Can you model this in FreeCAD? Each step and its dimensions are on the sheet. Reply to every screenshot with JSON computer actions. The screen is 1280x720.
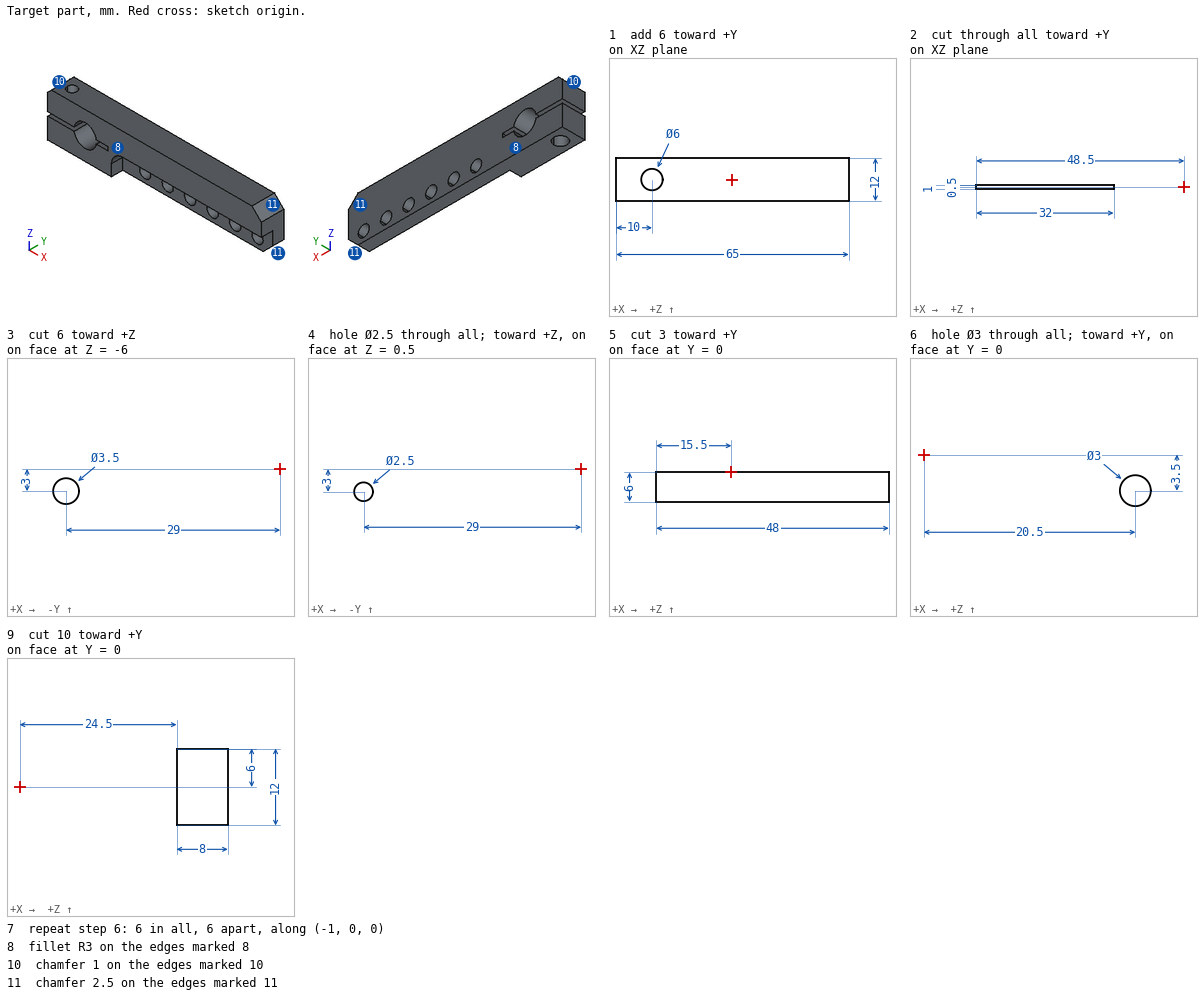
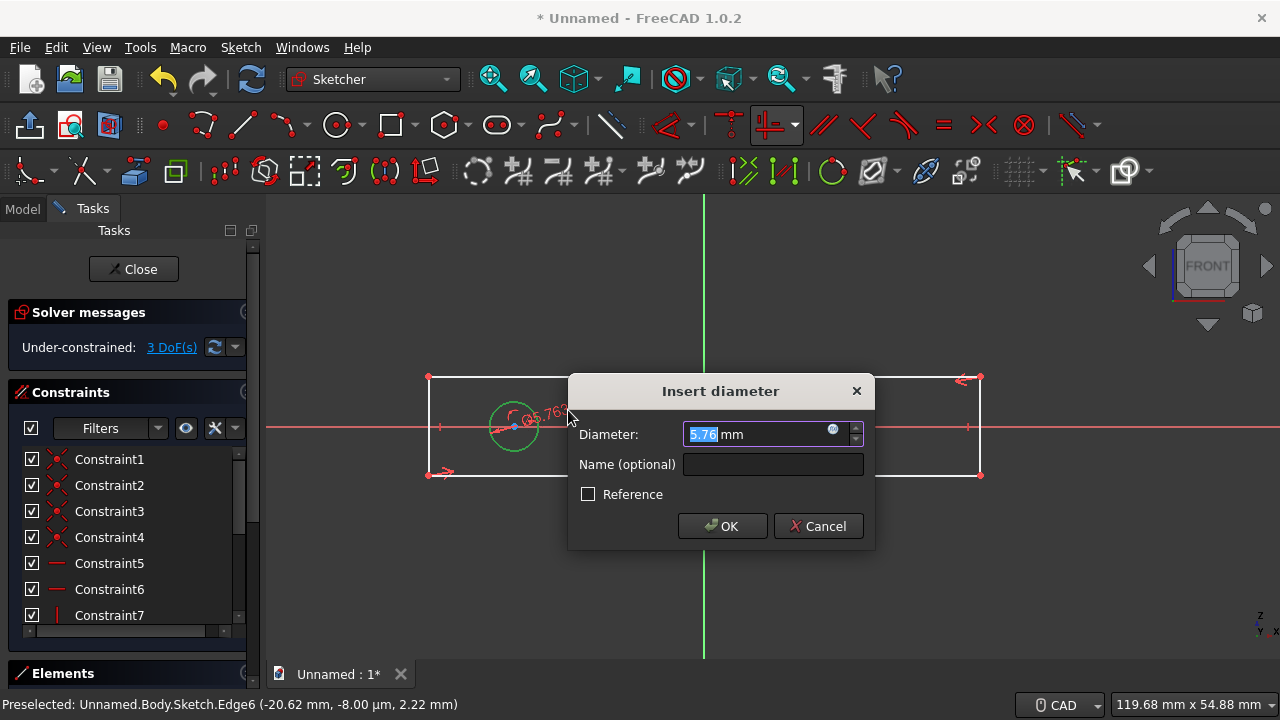
{"action": "type", "text": "6"}
{"action": "key", "text": "Return"}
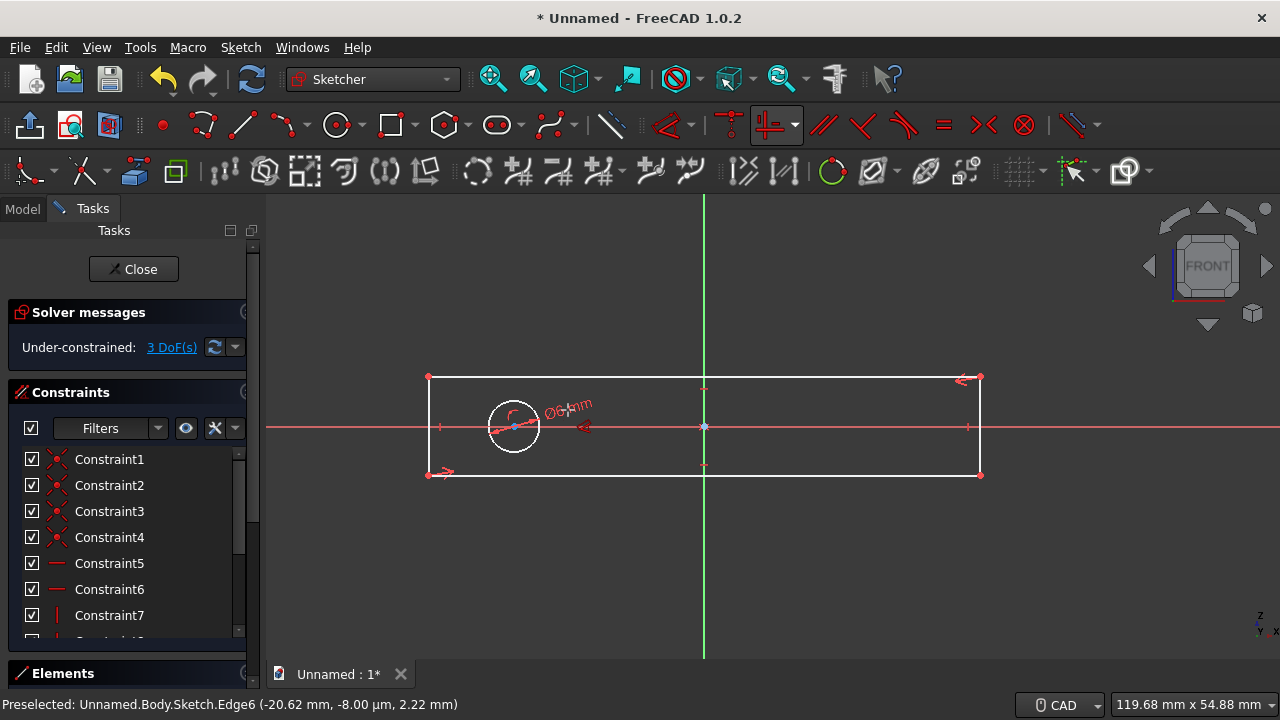
{"action": "left_click", "coordinate": [594, 476]}
{"action": "left_click", "coordinate": [577, 510]}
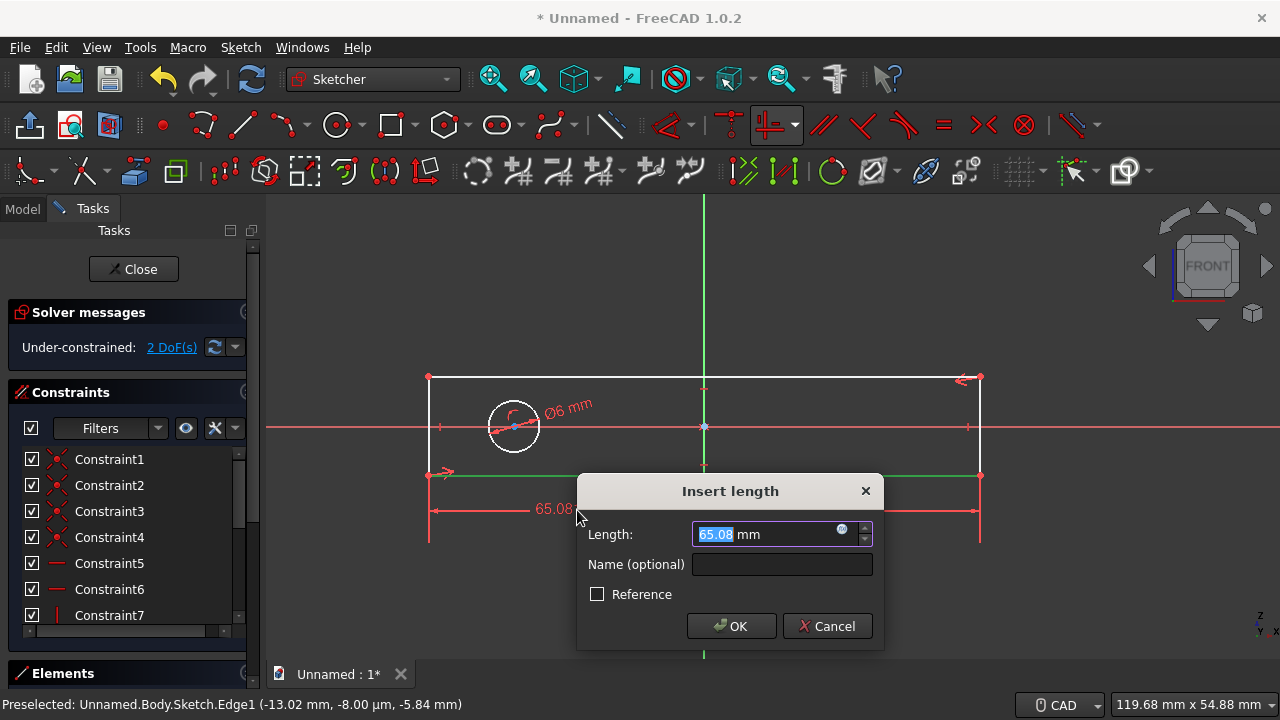
{"action": "type", "text": "65"}
{"action": "key", "text": "Return"}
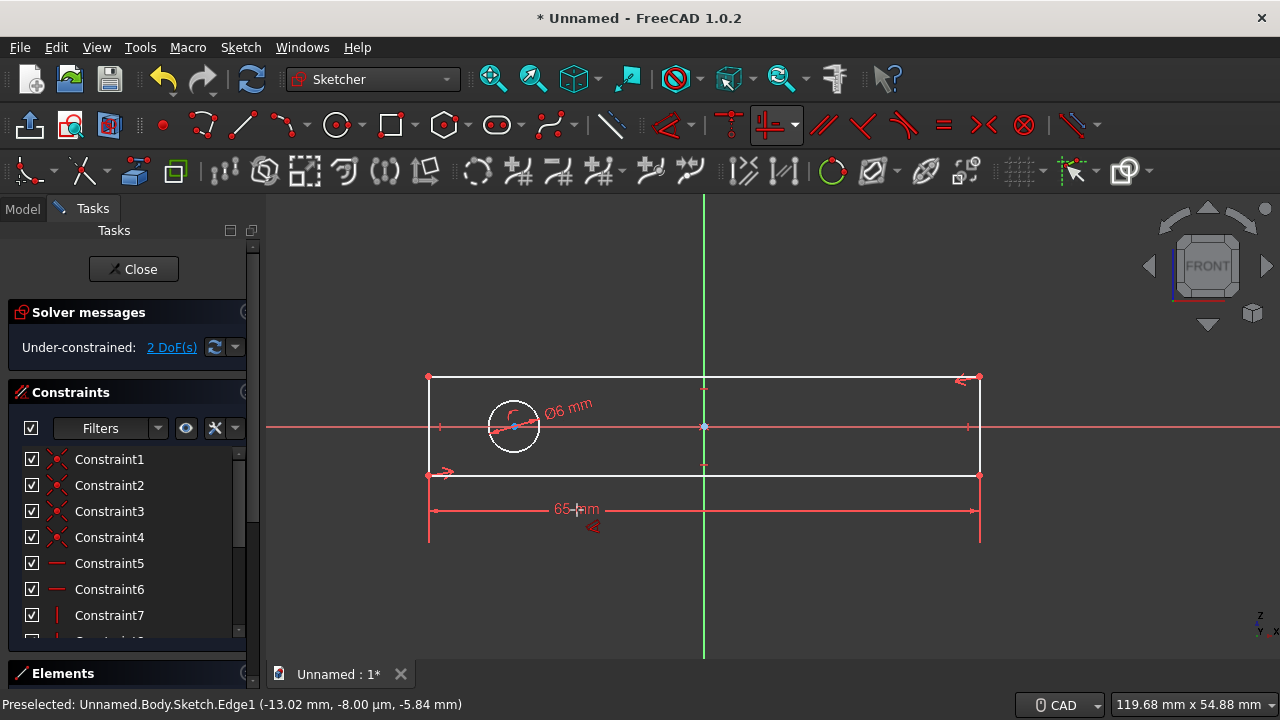
{"action": "left_click", "coordinate": [980, 446]}
{"action": "left_click", "coordinate": [1014, 404]}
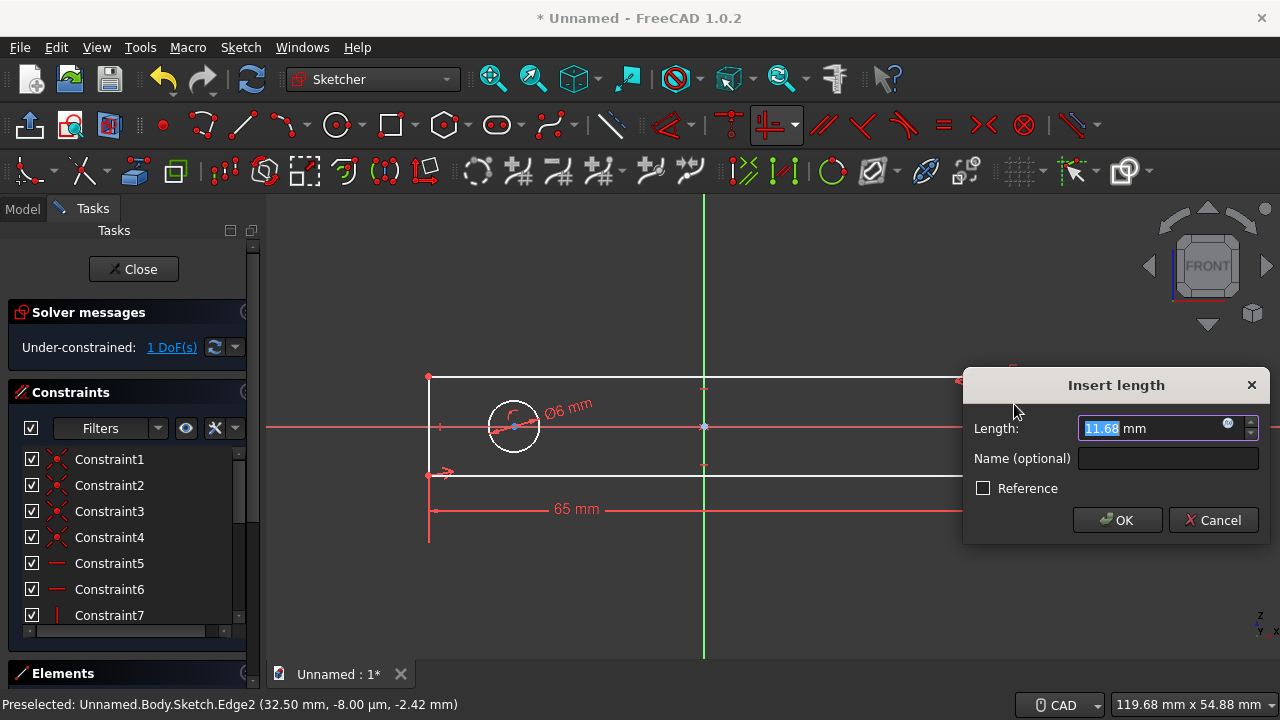
{"action": "type", "text": "12"}
{"action": "key", "text": "Return"}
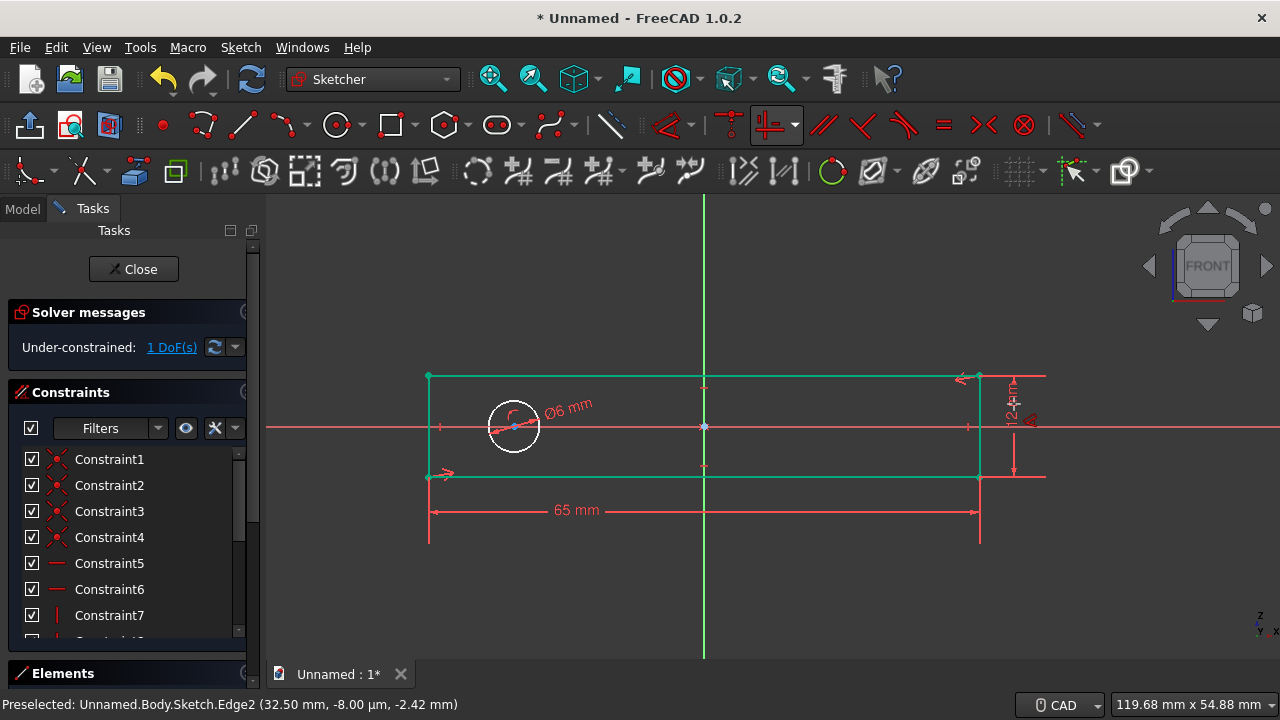
{"action": "left_click", "coordinate": [429, 477]}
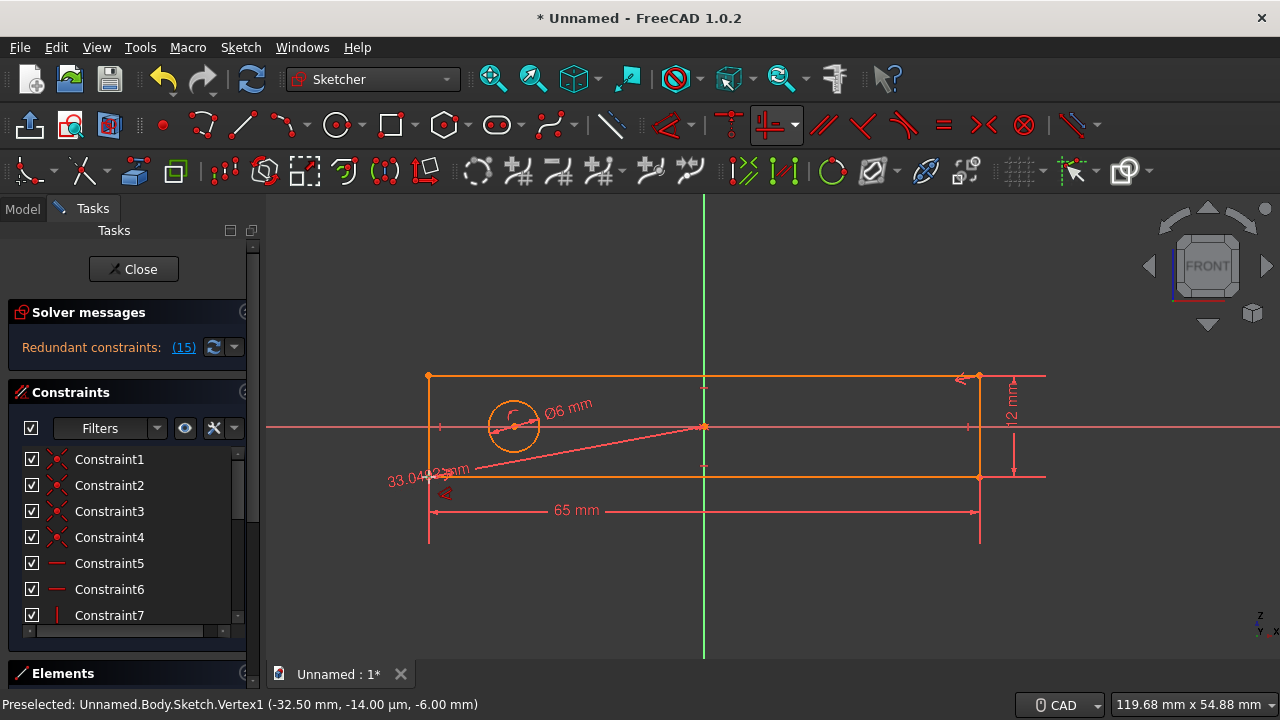
{"action": "left_click", "coordinate": [514, 426]}
{"action": "left_click", "coordinate": [471, 511]}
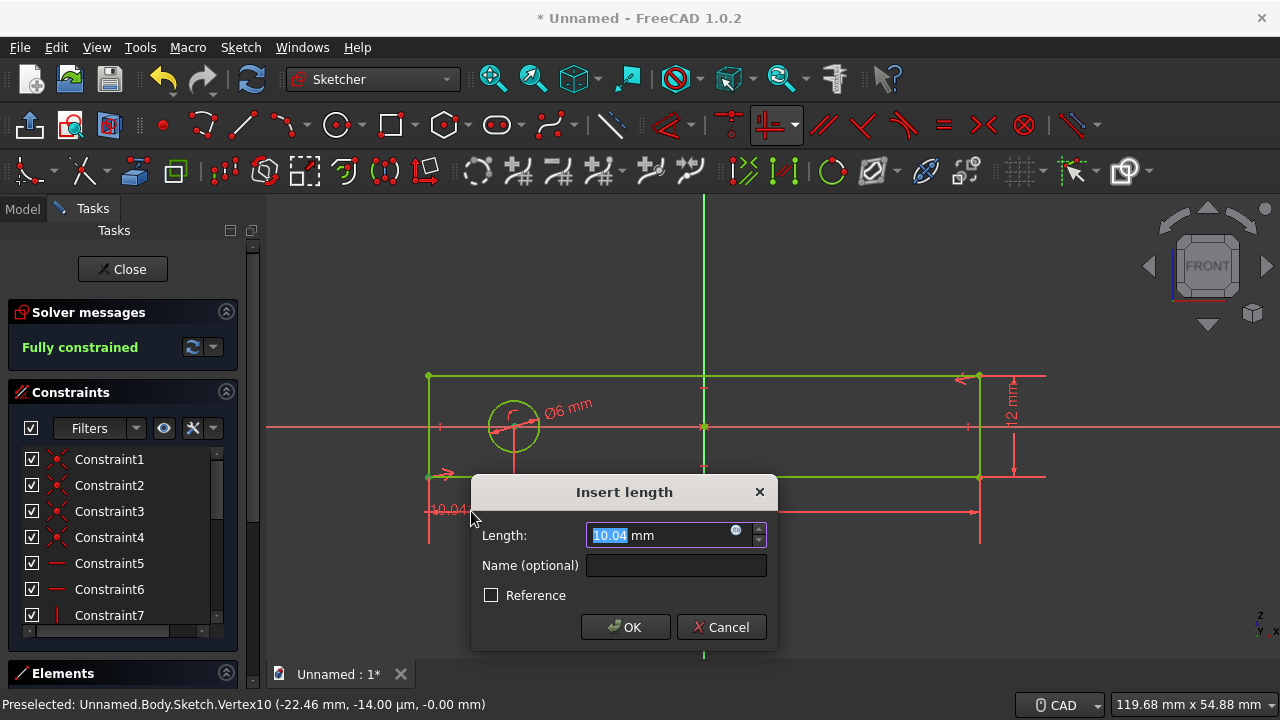
{"action": "type", "text": "10"}
{"action": "key", "text": "Return"}
{"action": "key", "text": "Escape"}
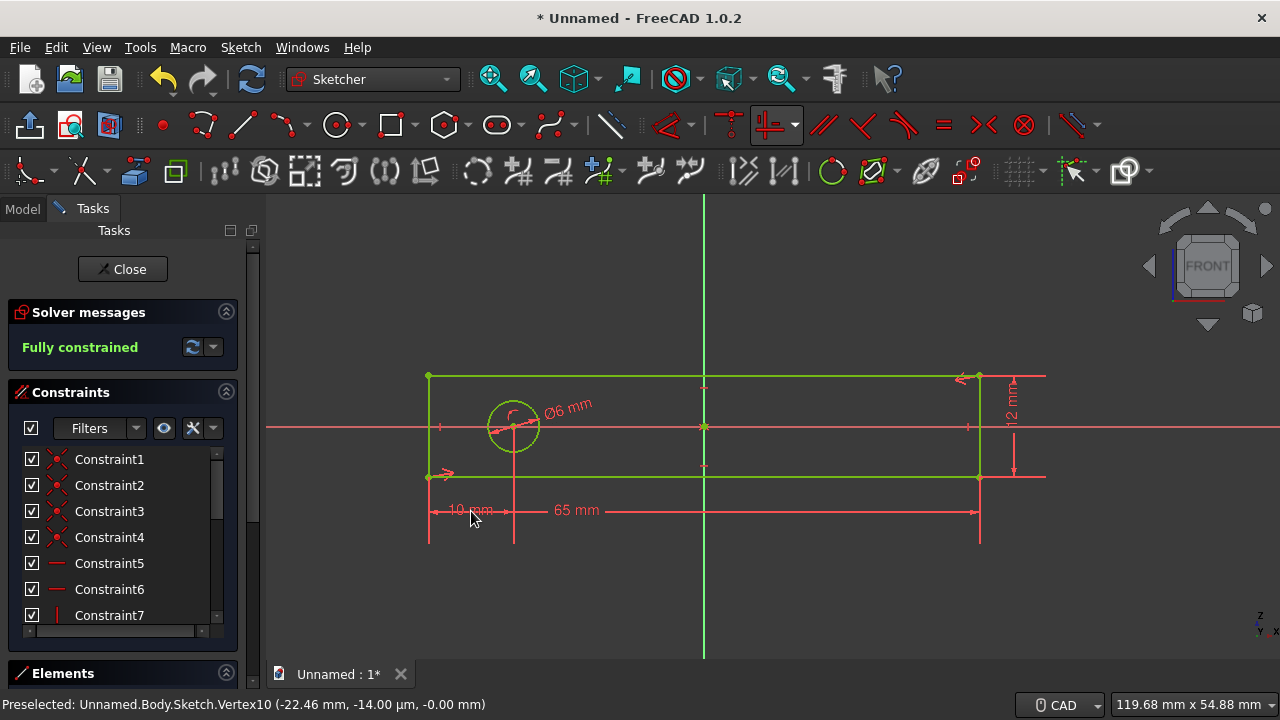
{"action": "left_click", "coordinate": [123, 269]}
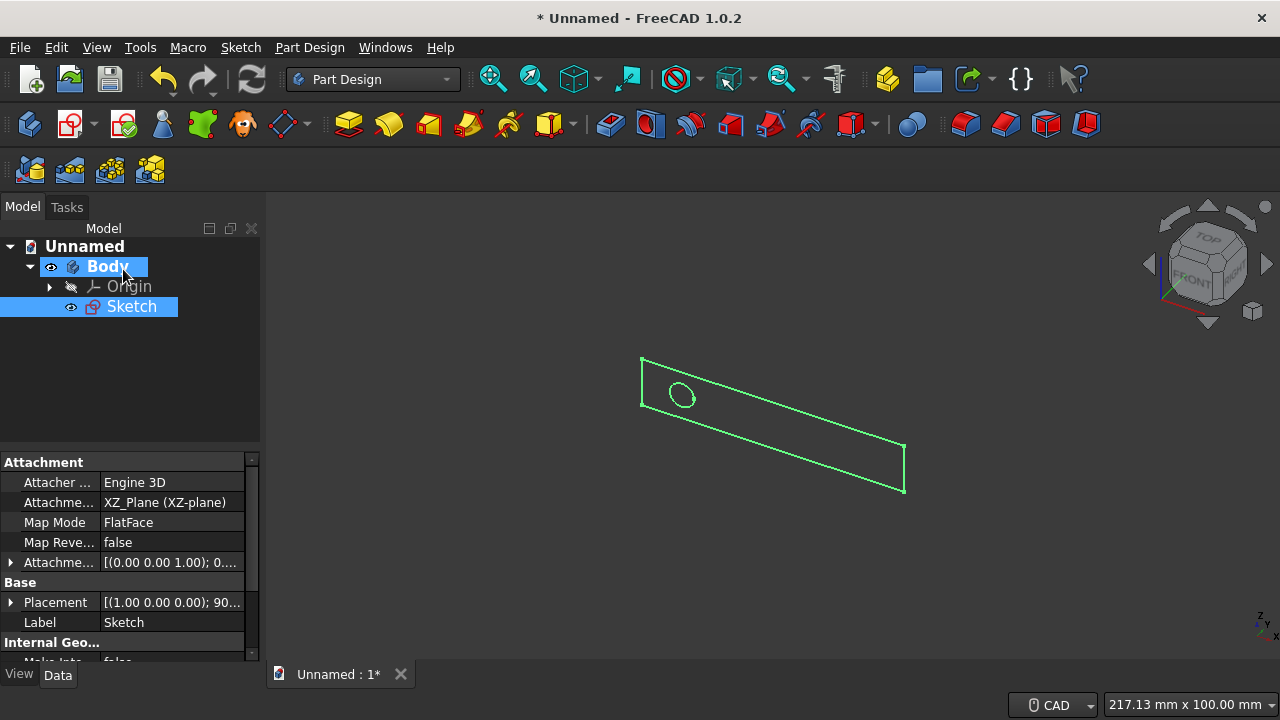
{"action": "left_click", "coordinate": [350, 124]}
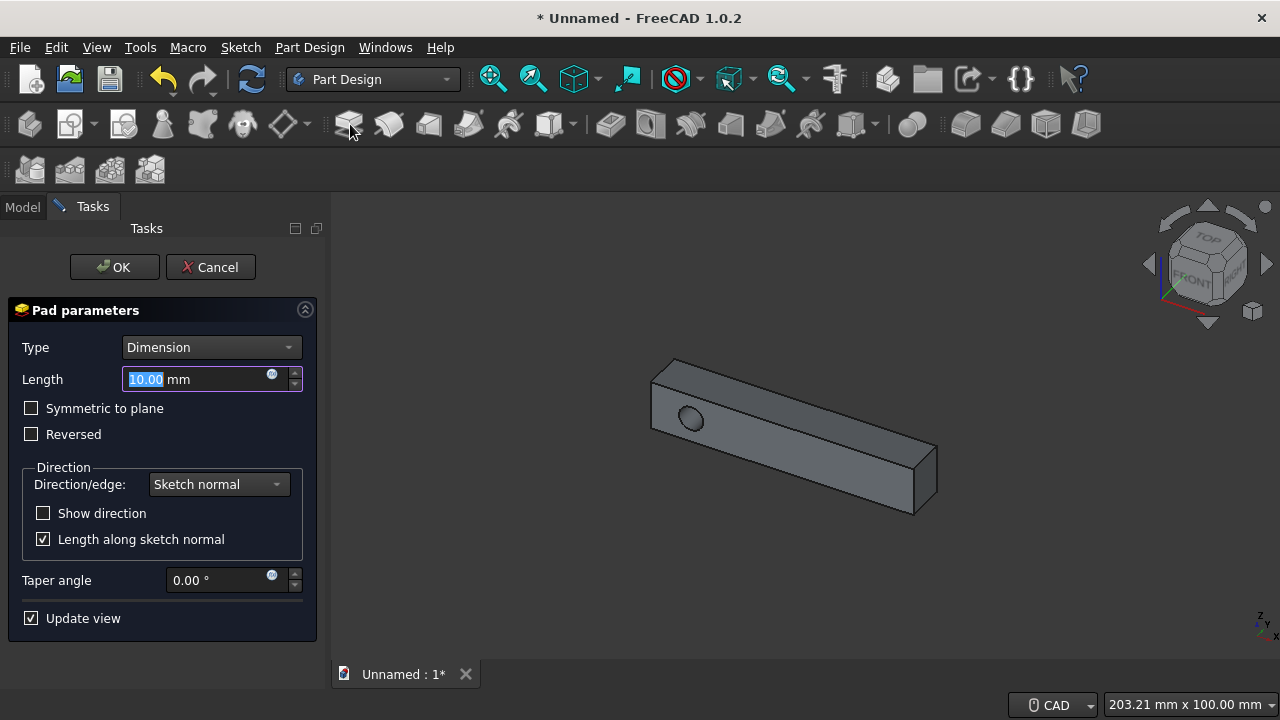
{"action": "type", "text": "6"}
{"action": "key", "text": "Tab"}